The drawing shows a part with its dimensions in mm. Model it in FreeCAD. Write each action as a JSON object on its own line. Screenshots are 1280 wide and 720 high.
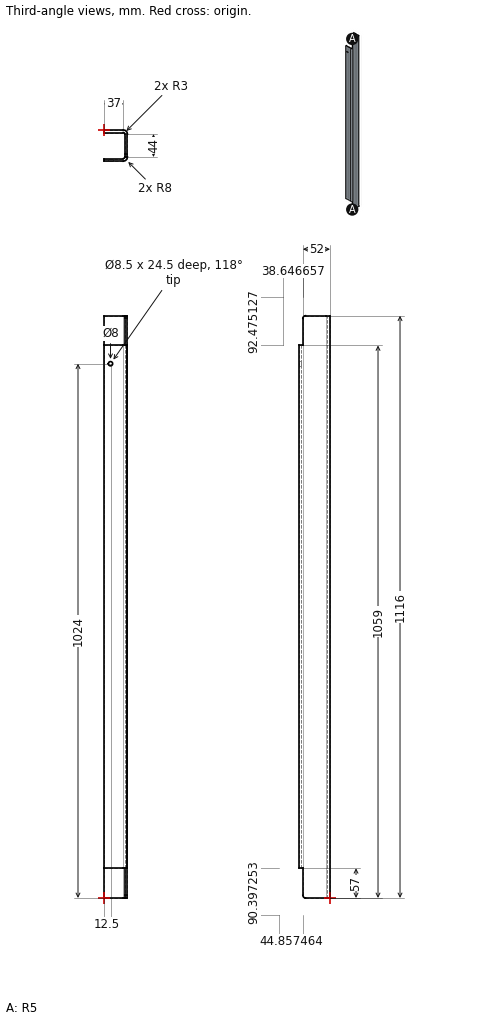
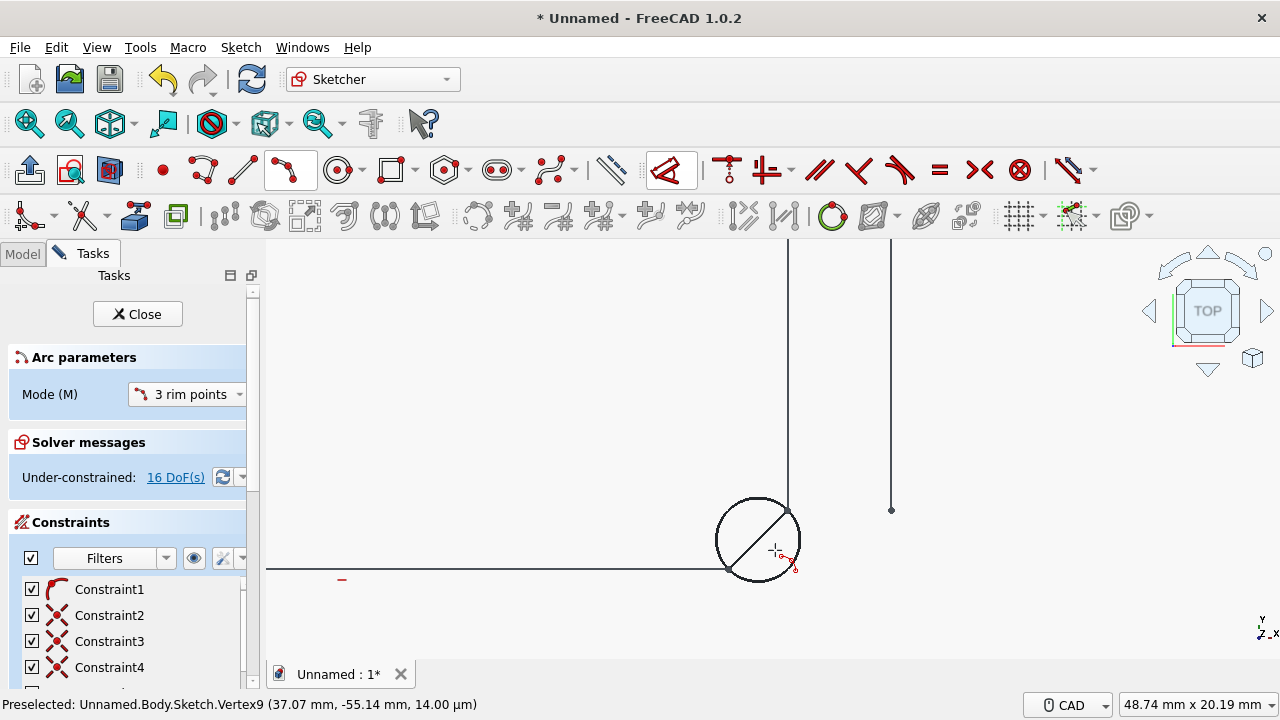
{"action": "left_click", "coordinate": [771, 548]}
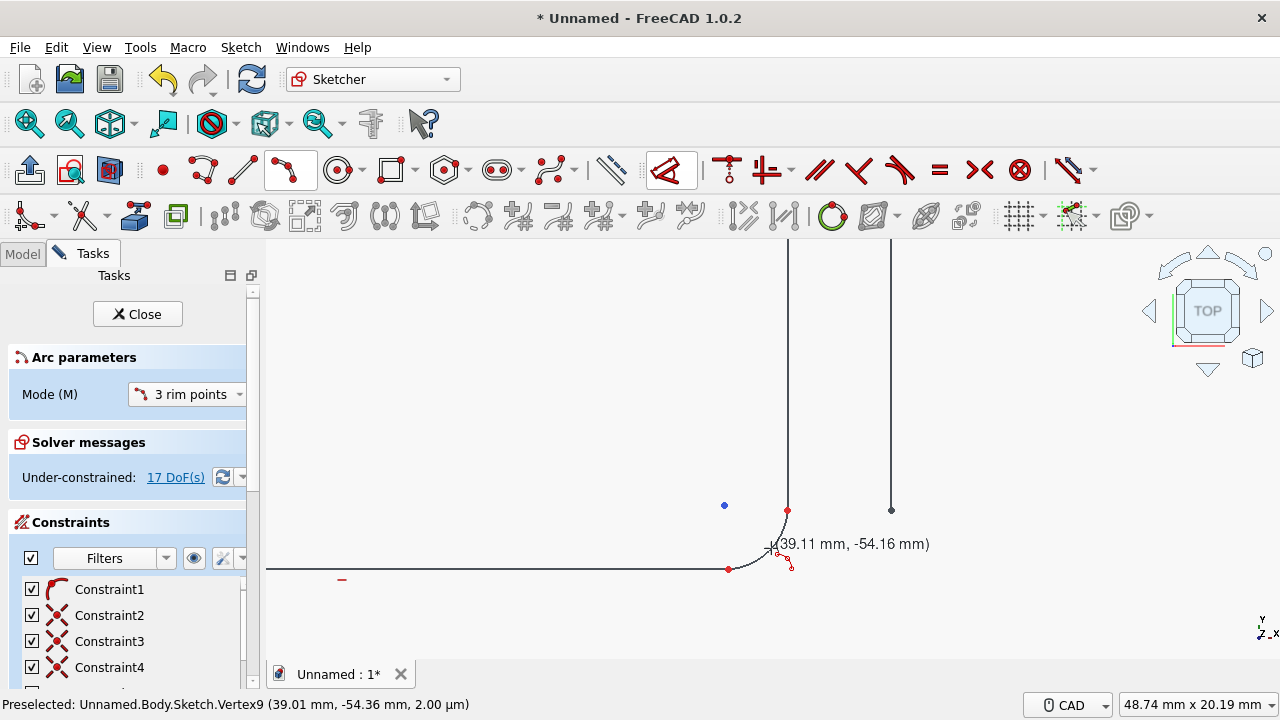
{"action": "scroll", "coordinate": [775, 551], "scroll_direction": "down", "scroll_amount": 8}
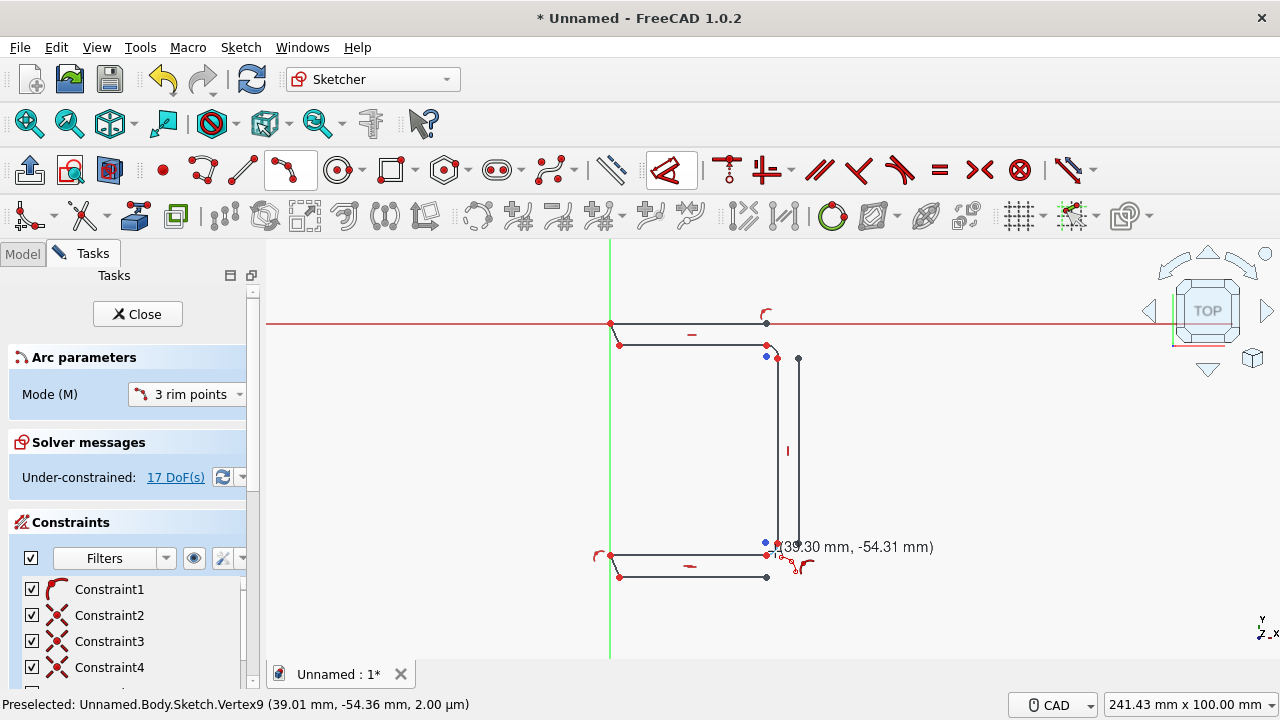
{"action": "left_click", "coordinate": [766, 577]}
{"action": "left_click", "coordinate": [799, 543]}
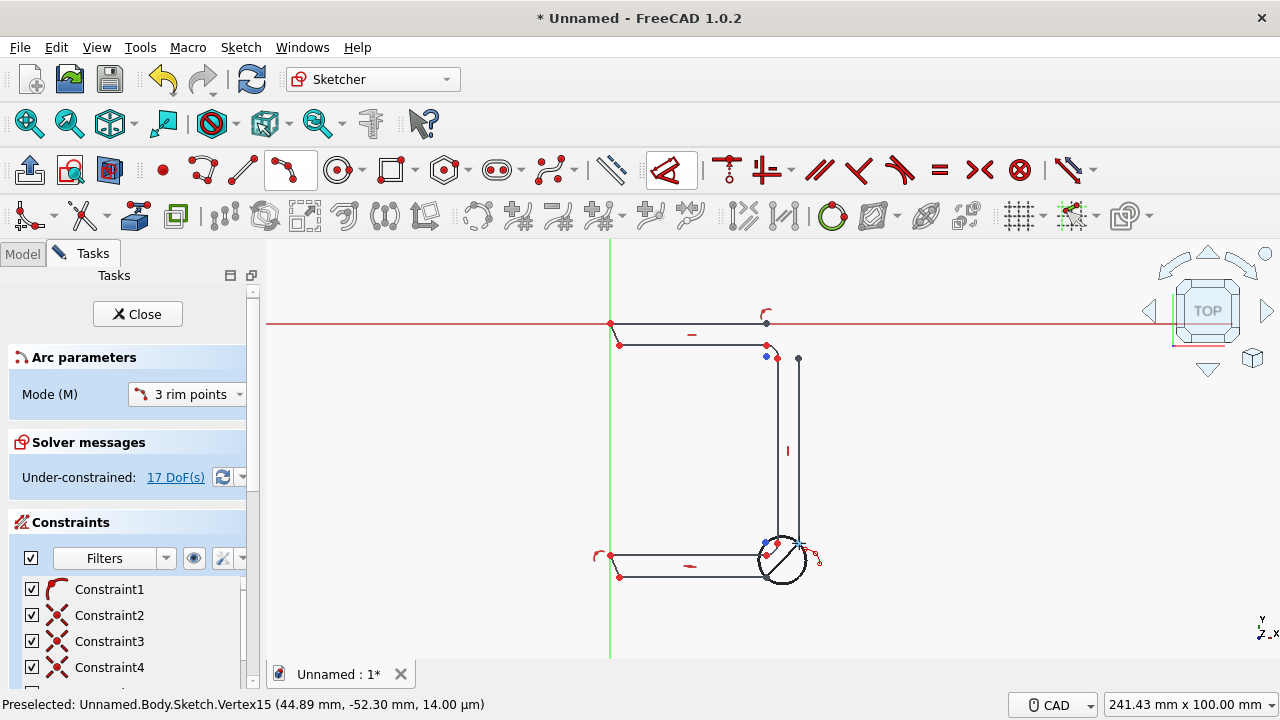
{"action": "scroll", "coordinate": [789, 566], "scroll_direction": "up", "scroll_amount": 3}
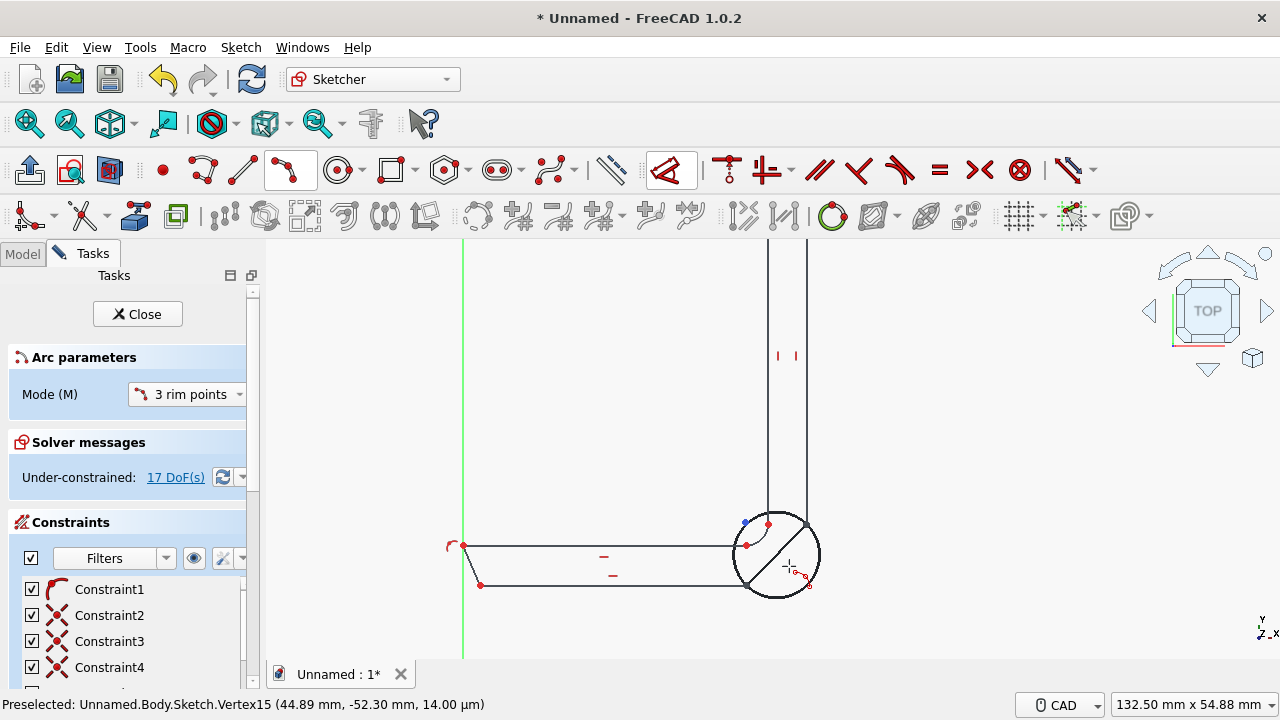
{"action": "left_click", "coordinate": [789, 565]}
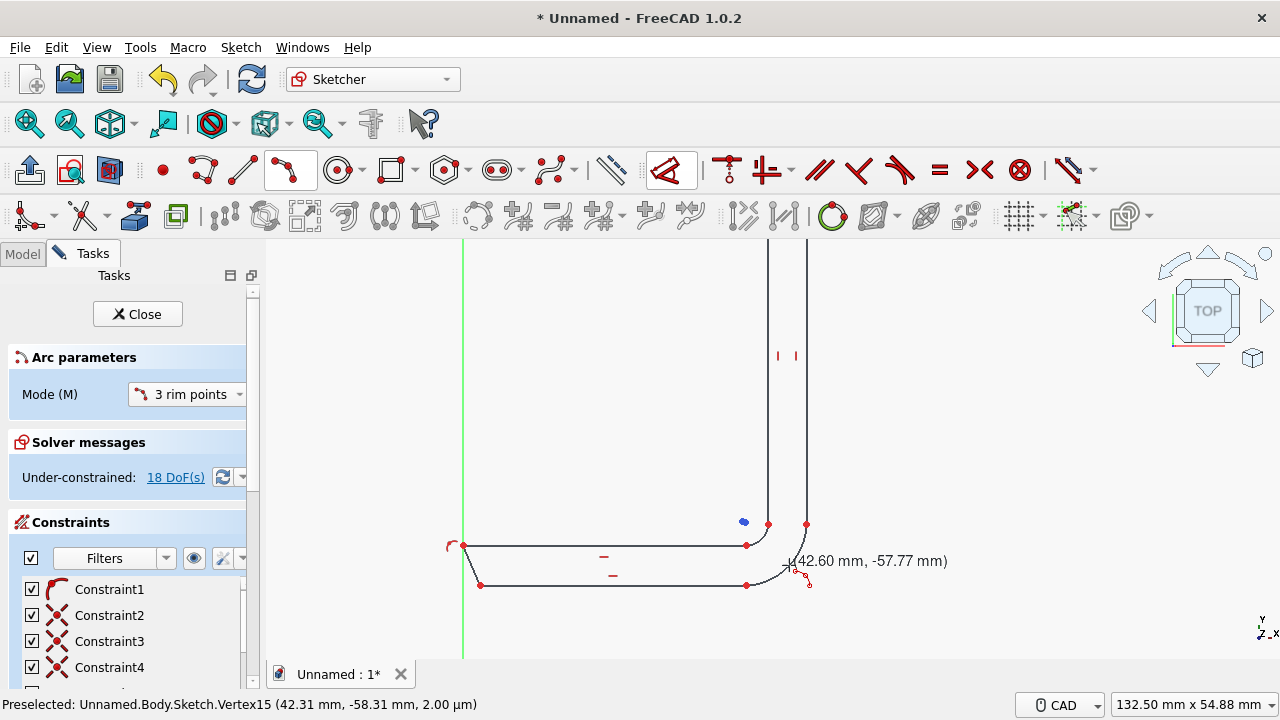
{"action": "scroll", "coordinate": [789, 565], "scroll_direction": "down", "scroll_amount": 3}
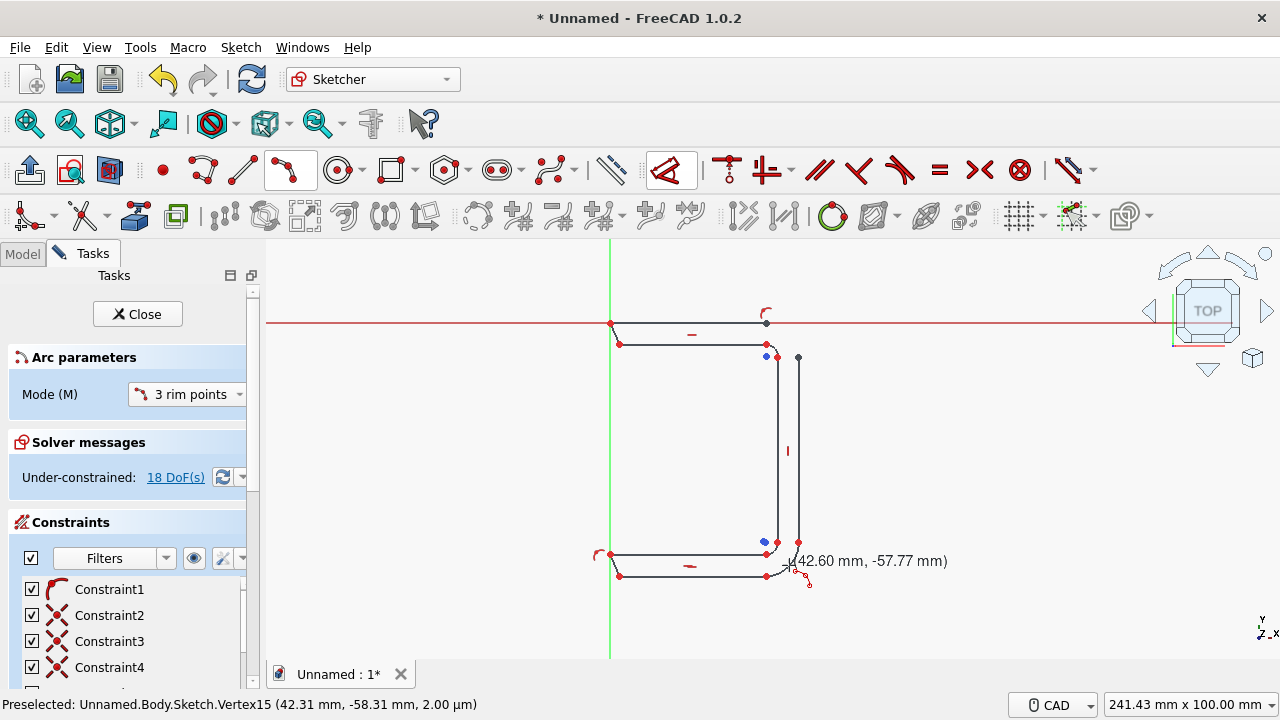
{"action": "left_click", "coordinate": [799, 358]}
{"action": "left_click", "coordinate": [766, 323]}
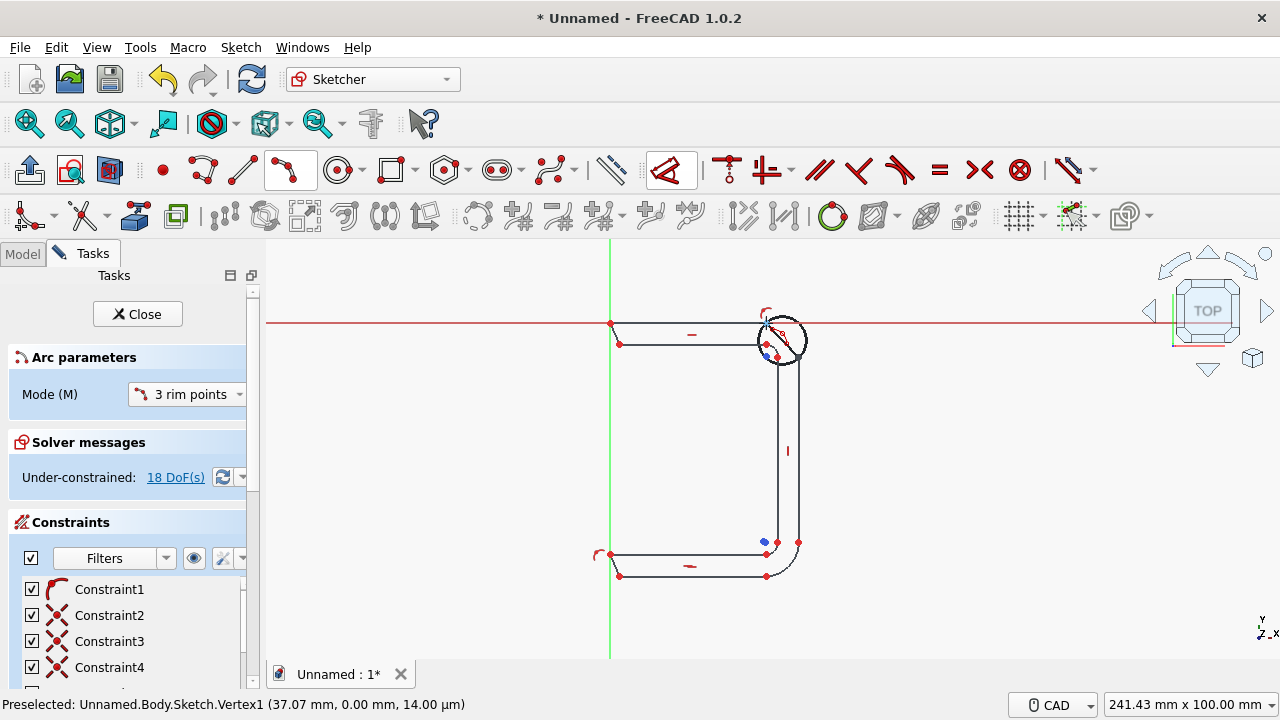
{"action": "scroll", "coordinate": [789, 333], "scroll_direction": "up", "scroll_amount": 3}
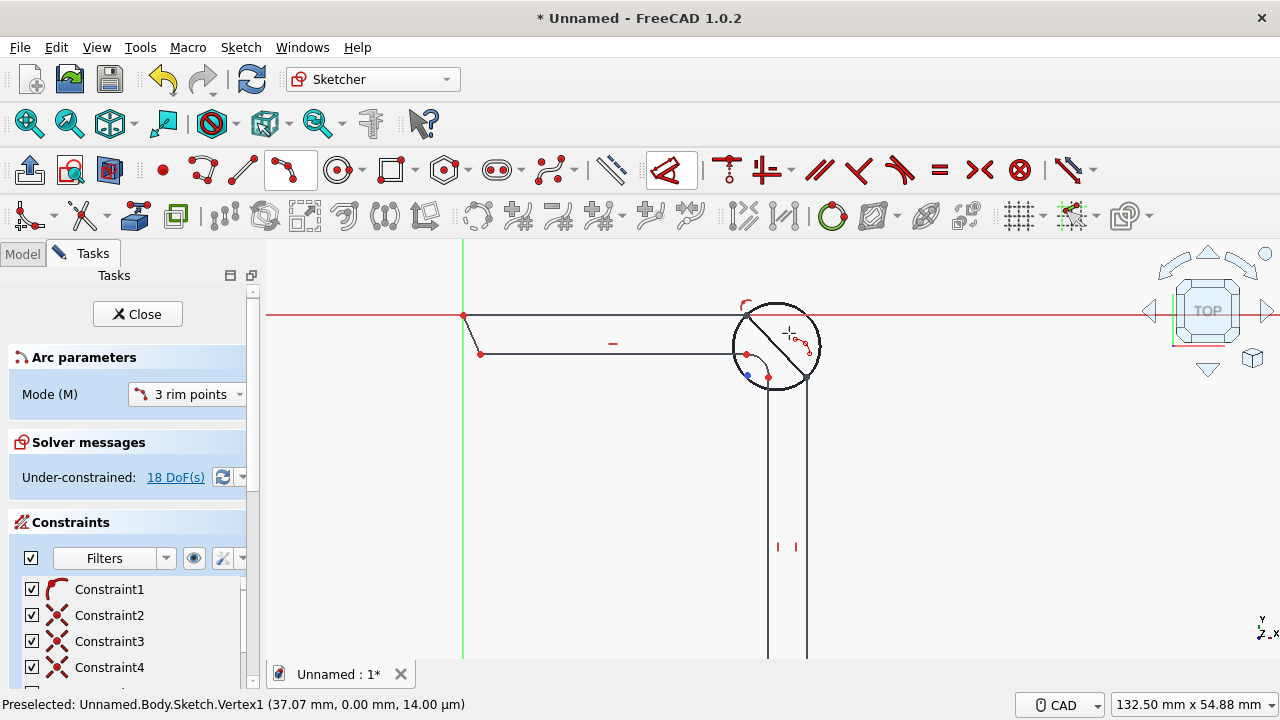
{"action": "left_click", "coordinate": [789, 333]}
{"action": "key", "text": "Escape"}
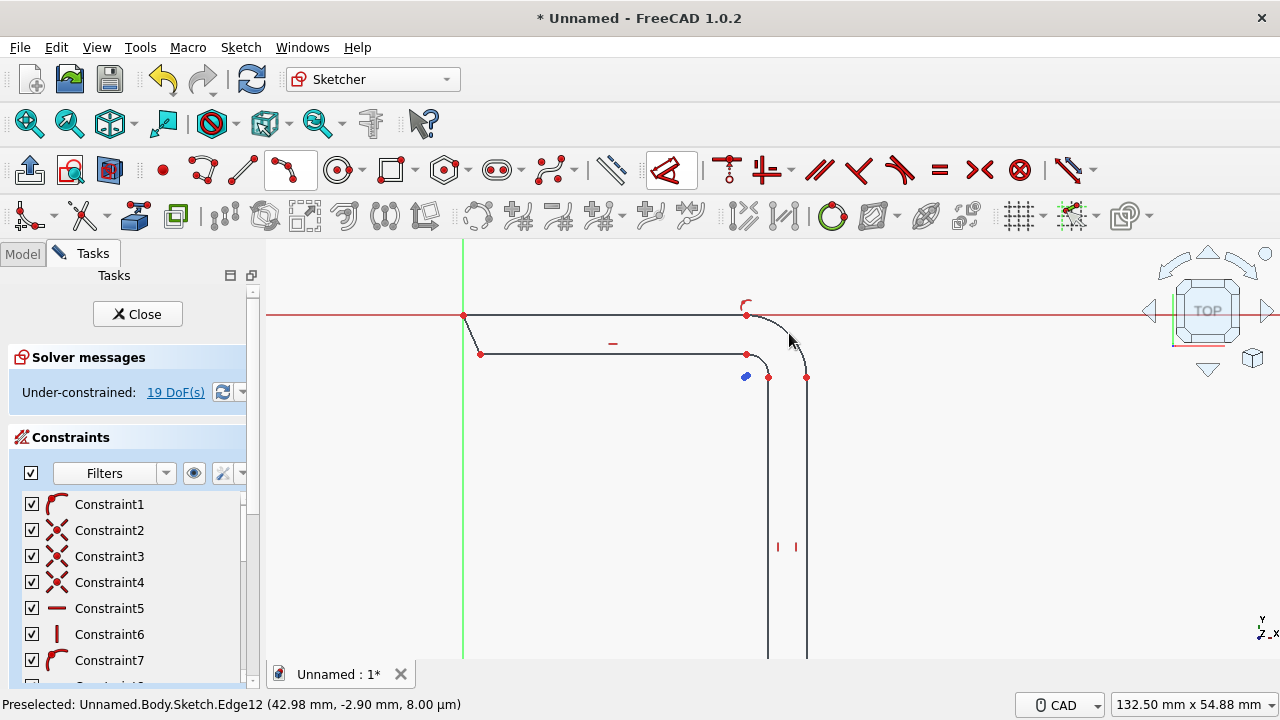
{"action": "left_click", "coordinate": [662, 315]}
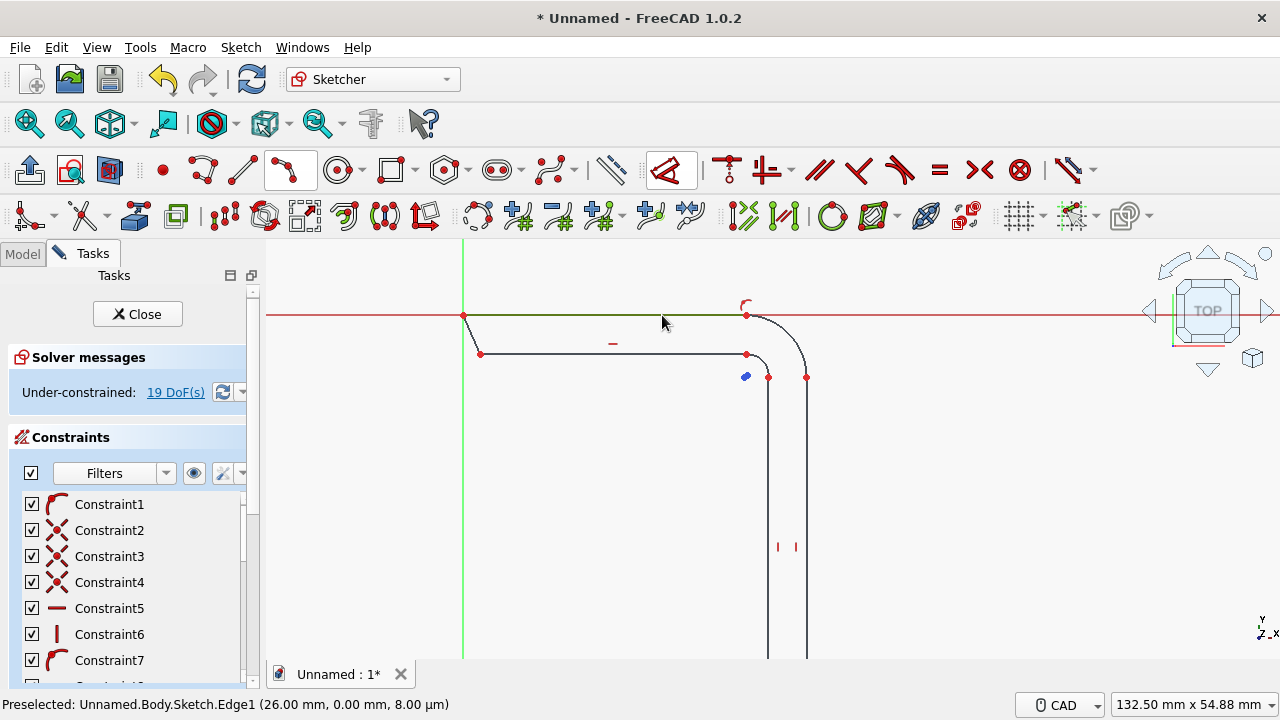
{"action": "left_click", "coordinate": [800, 350]}